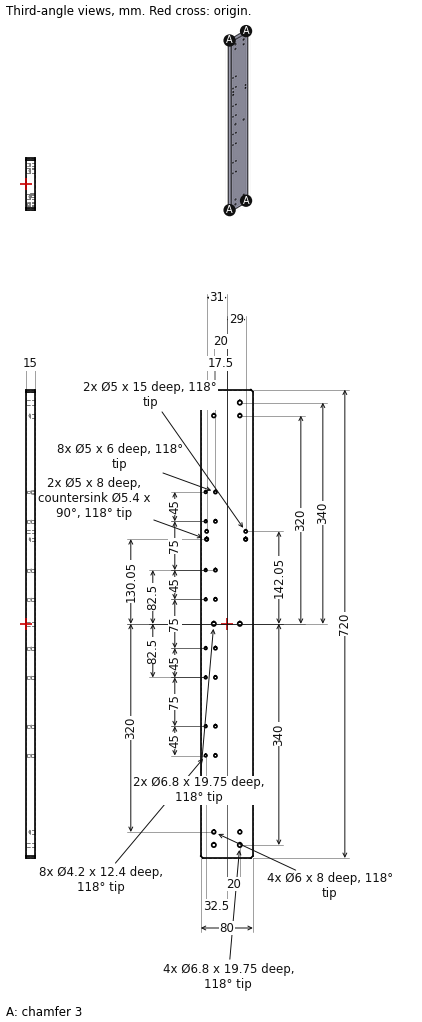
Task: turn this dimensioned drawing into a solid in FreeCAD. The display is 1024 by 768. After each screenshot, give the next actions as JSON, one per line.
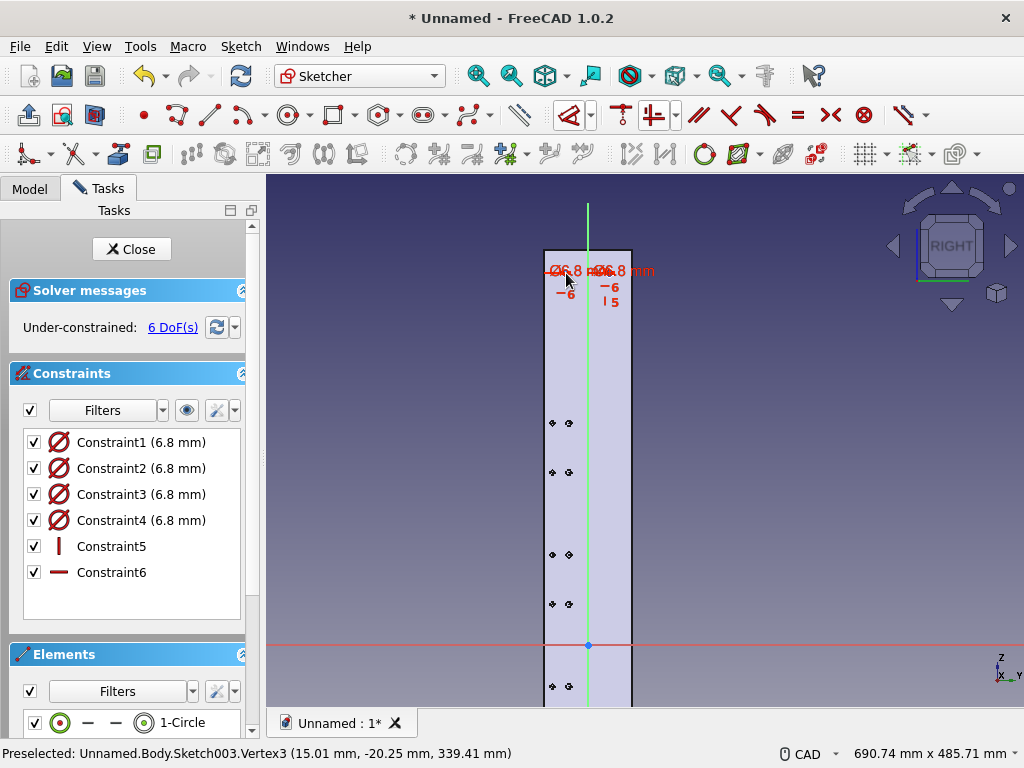
{"action": "left_click", "coordinate": [566, 273]}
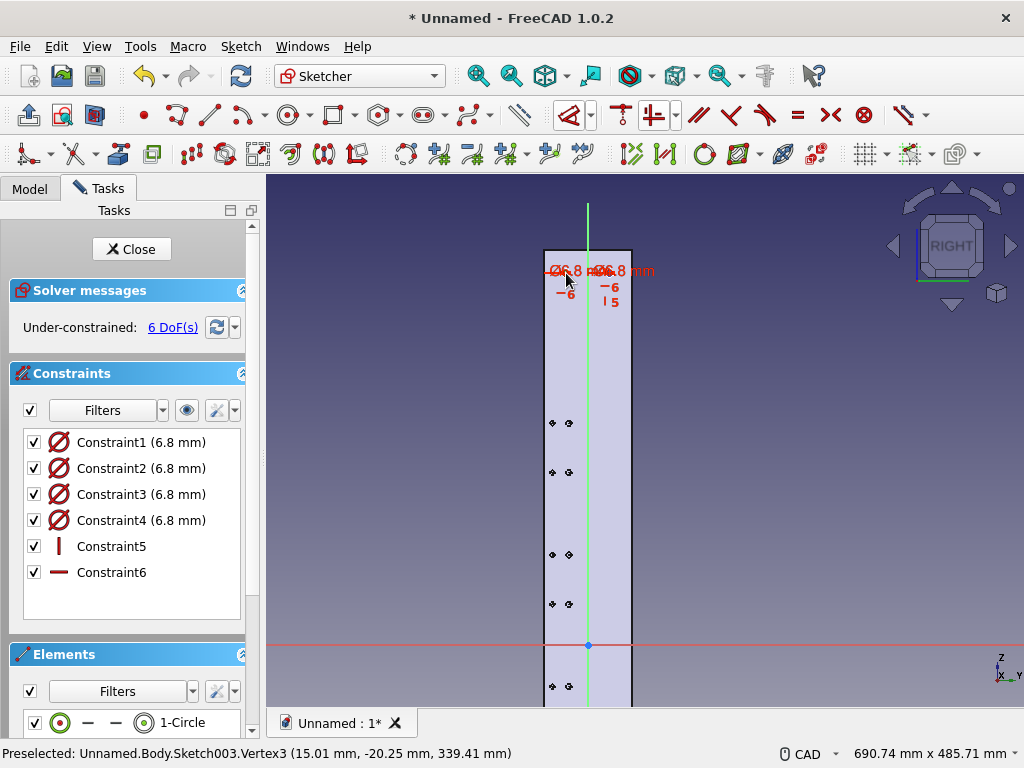
{"action": "scroll", "coordinate": [567, 273], "scroll_direction": "down", "scroll_amount": 4}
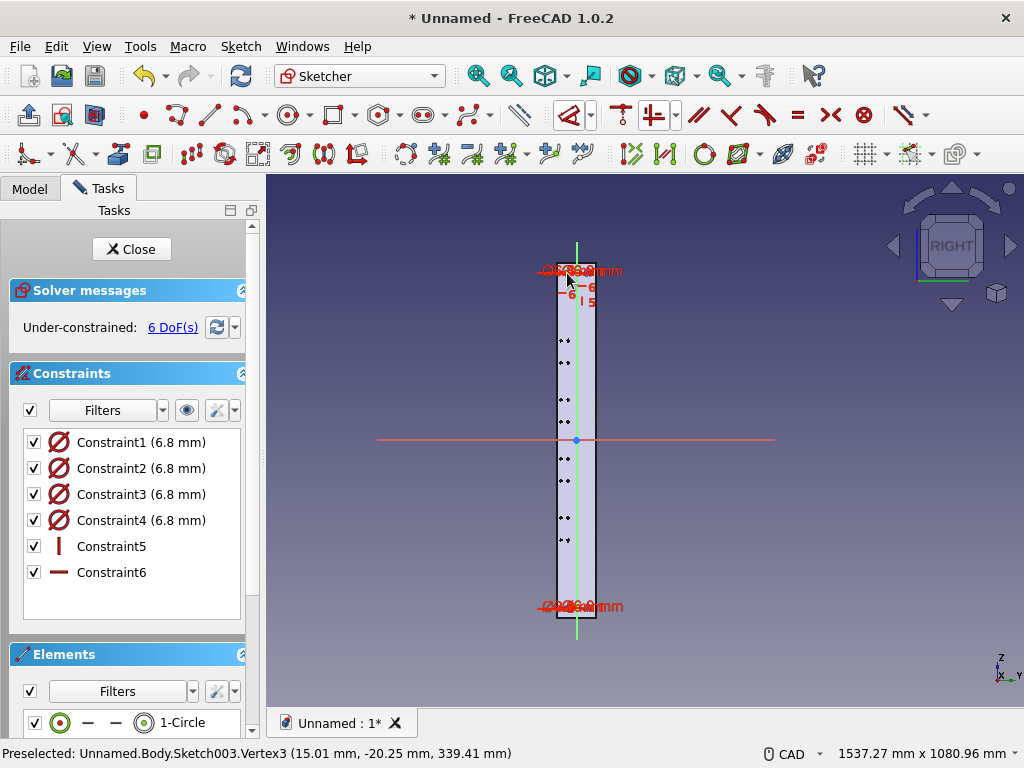
{"action": "left_click", "coordinate": [567, 609]}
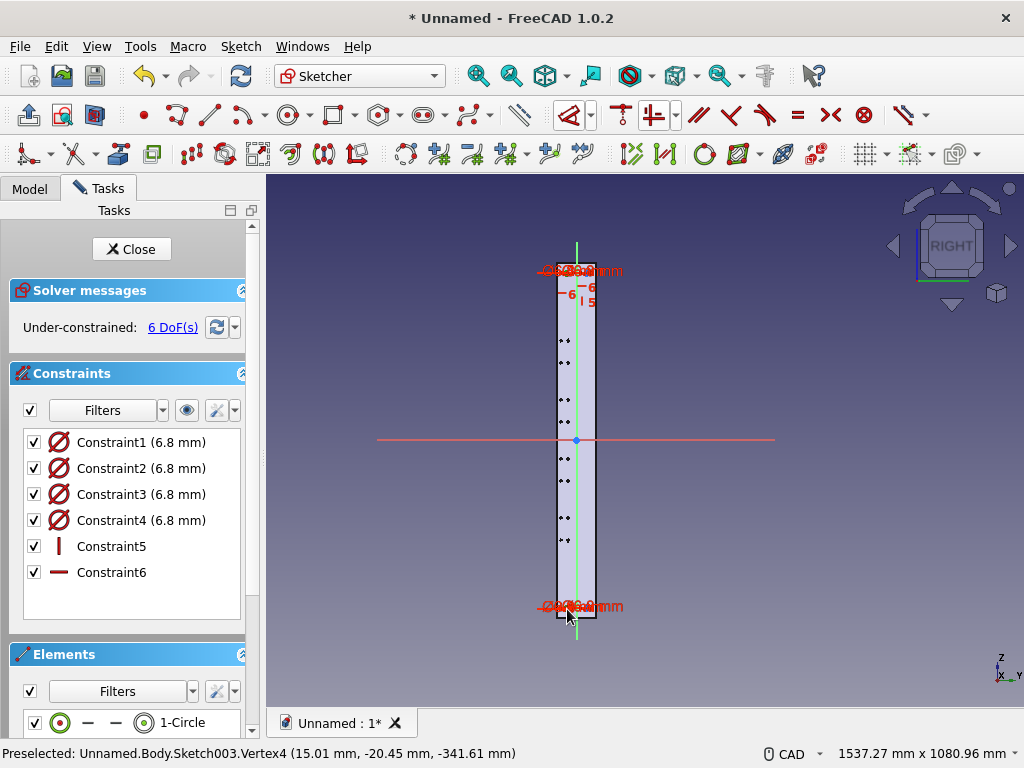
{"action": "left_click", "coordinate": [676, 116]}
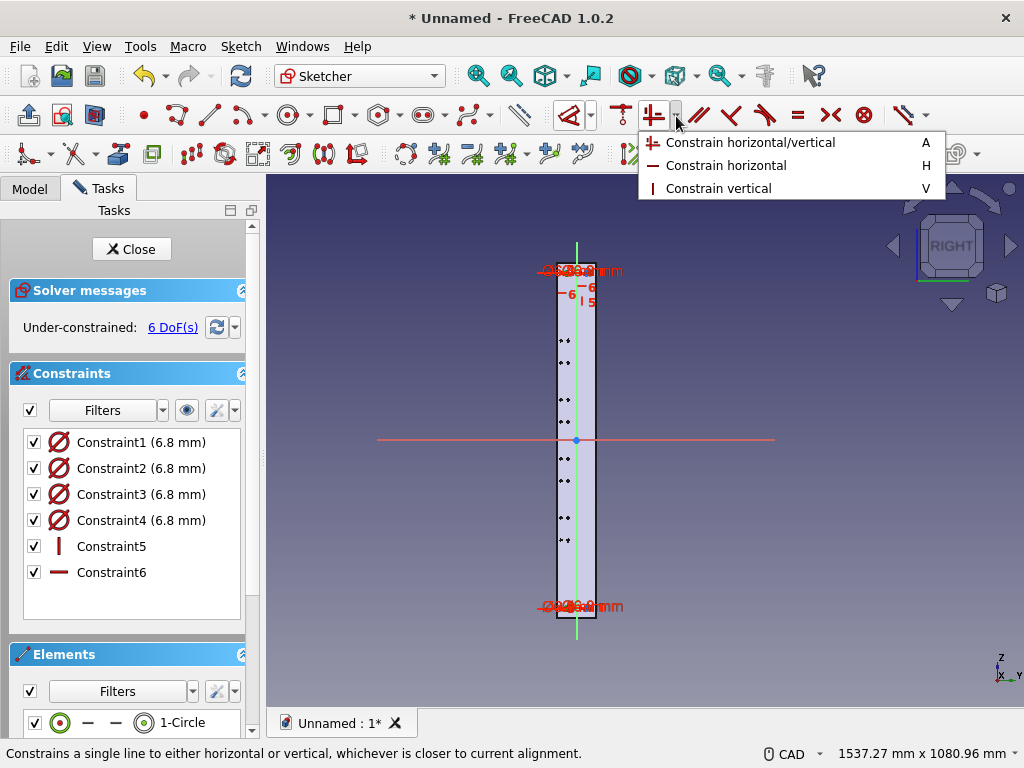
{"action": "left_click", "coordinate": [792, 188]}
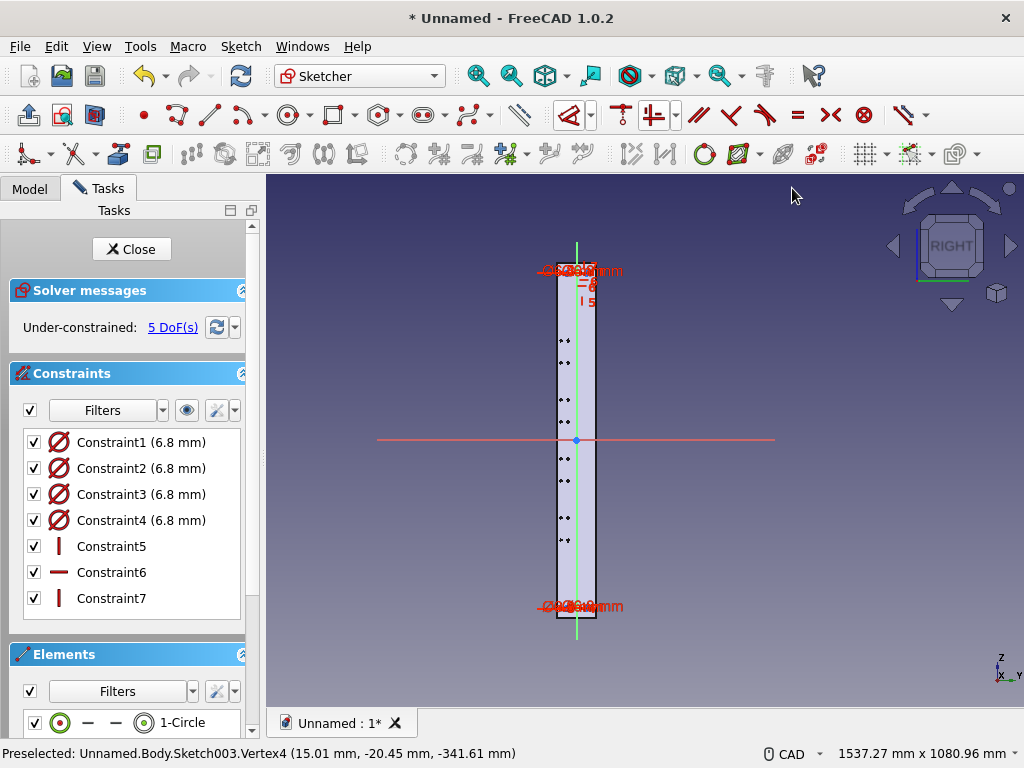
{"action": "scroll", "coordinate": [586, 608], "scroll_direction": "up", "scroll_amount": 4}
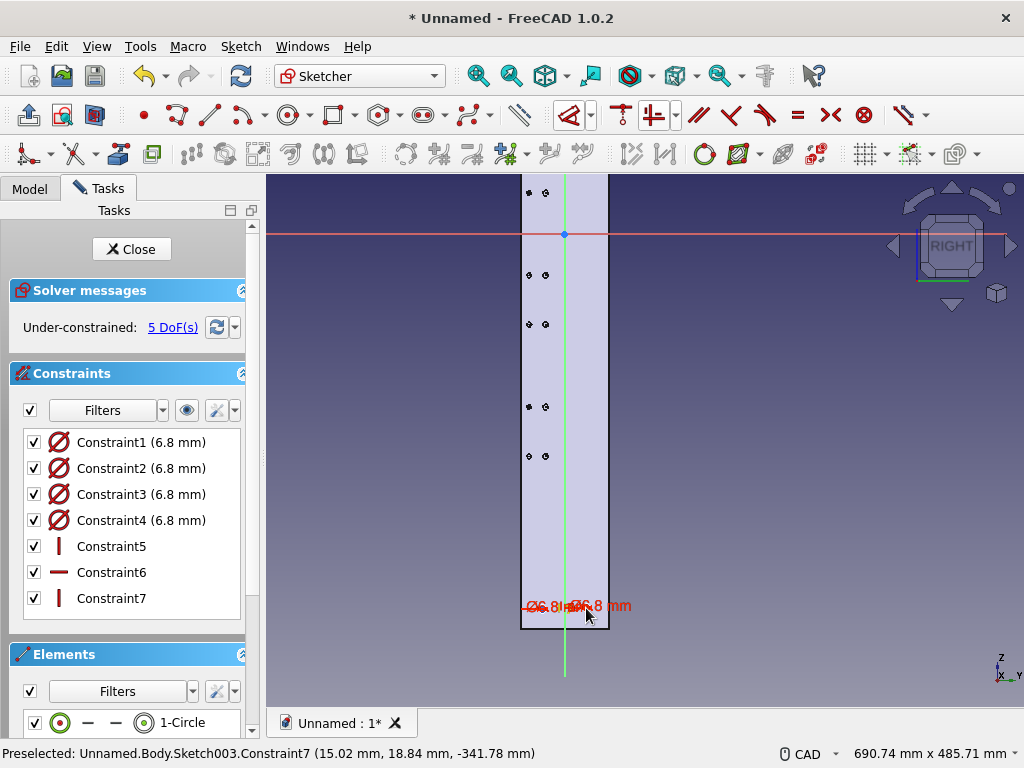
{"action": "left_click", "coordinate": [586, 608]}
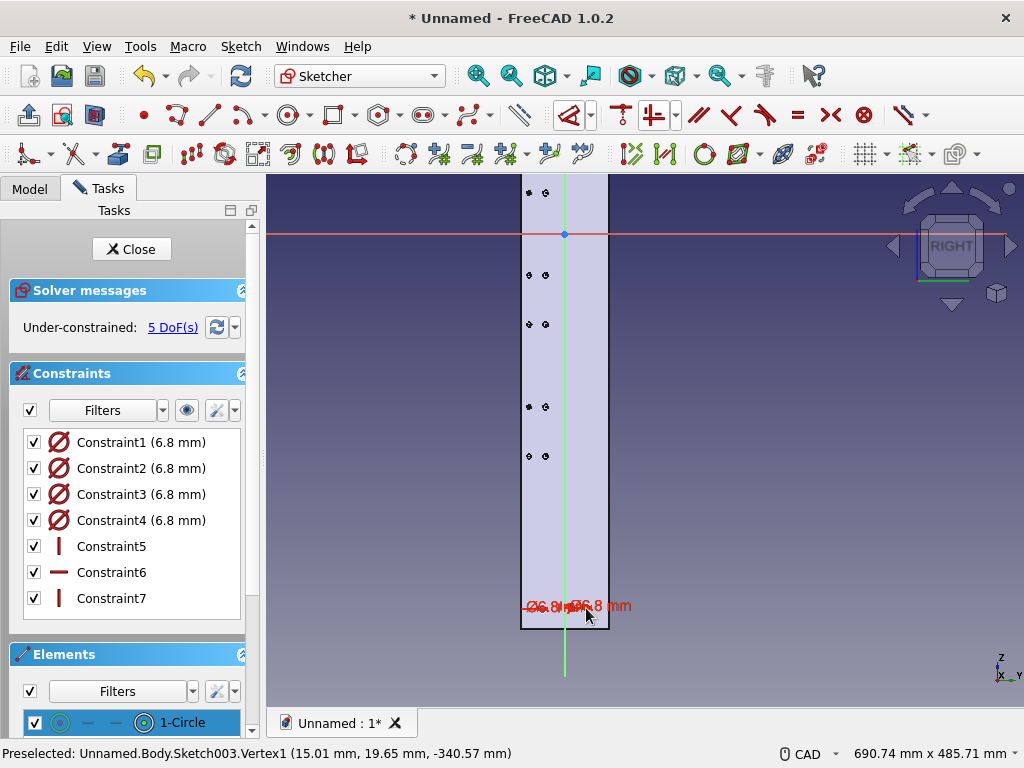
{"action": "left_click", "coordinate": [543, 609]}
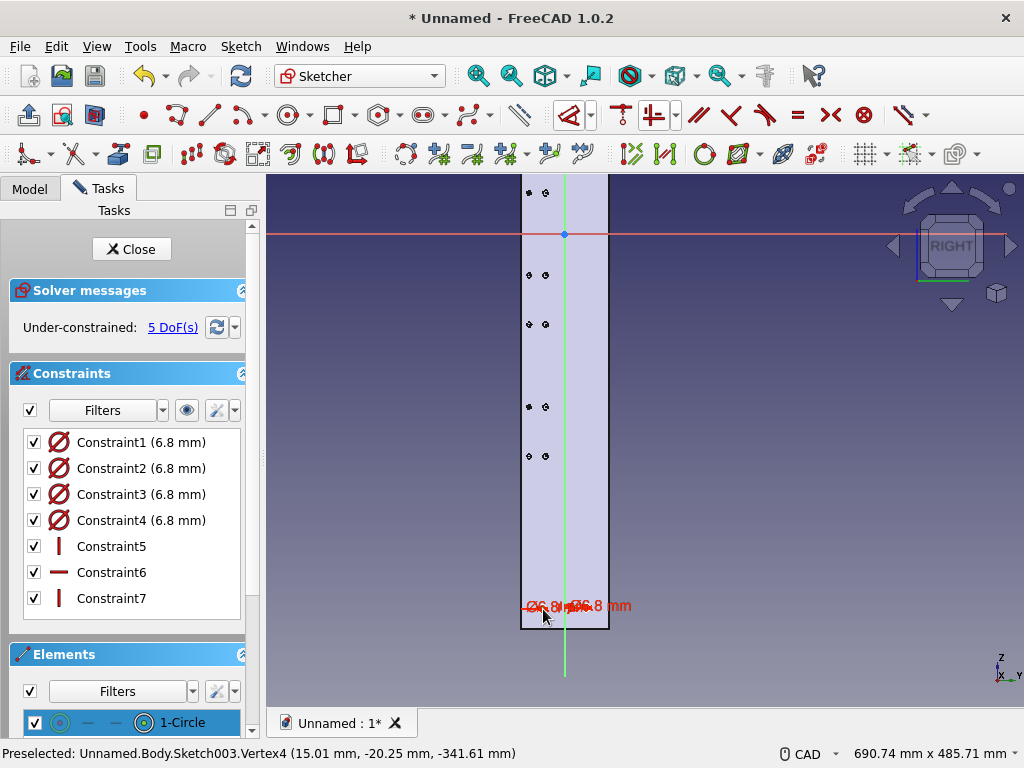
{"action": "left_click", "coordinate": [676, 116]}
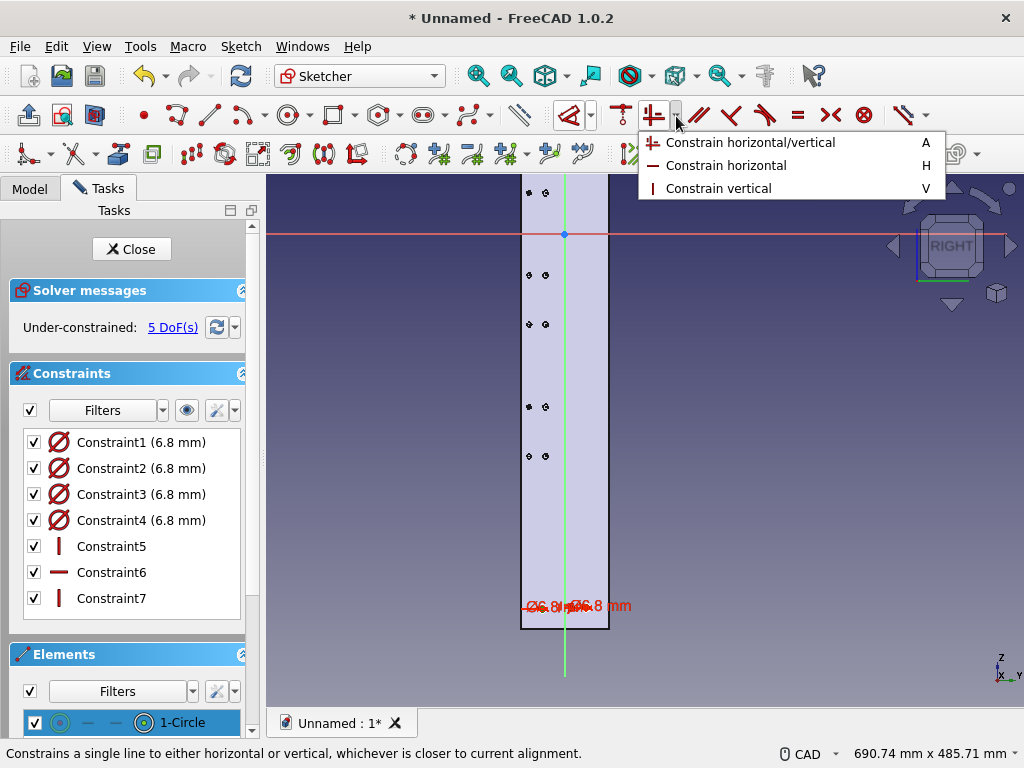
{"action": "left_click", "coordinate": [792, 166]}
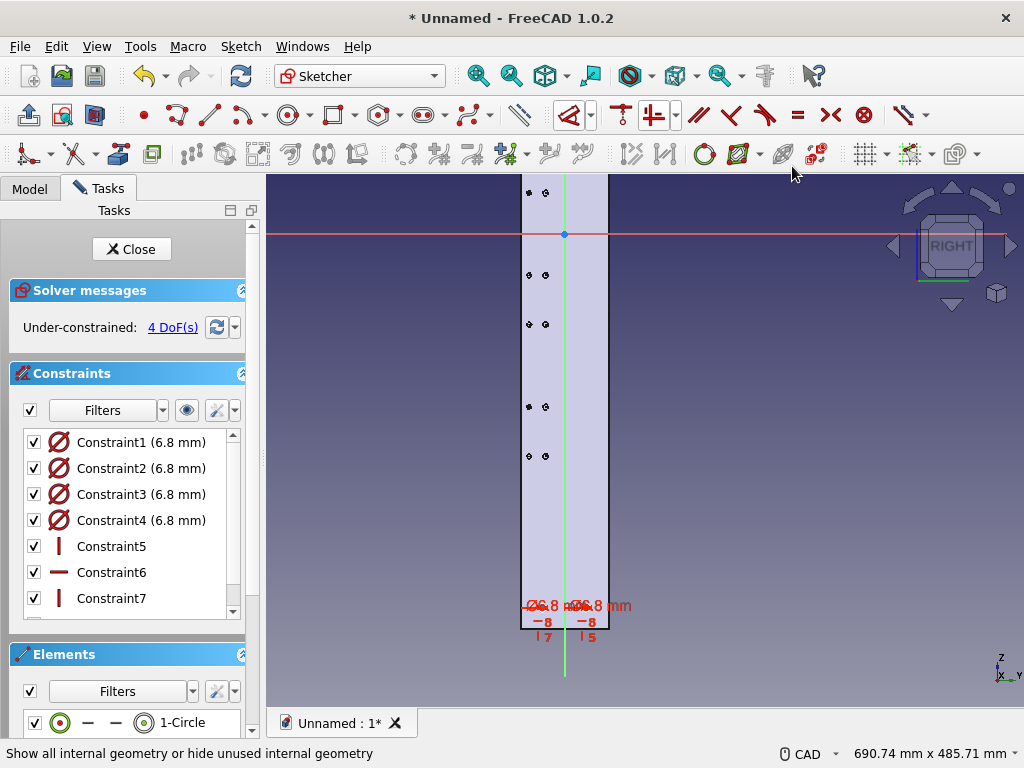
{"action": "scroll", "coordinate": [586, 608], "scroll_direction": "up", "scroll_amount": 3}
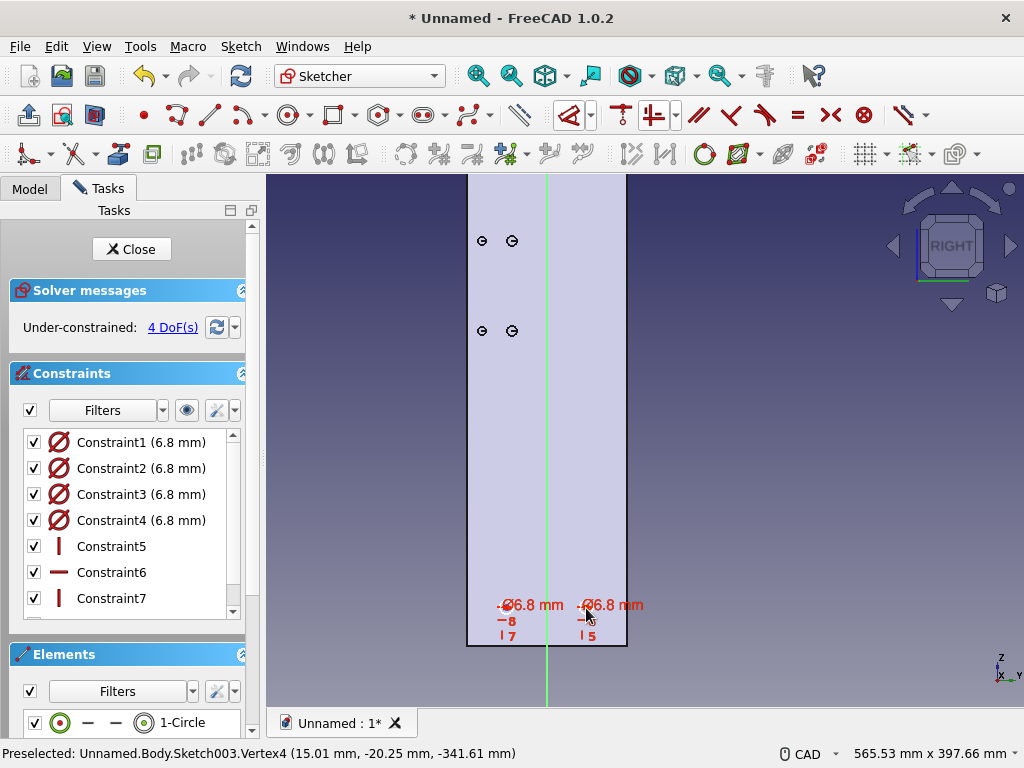
{"action": "left_click", "coordinate": [586, 607]}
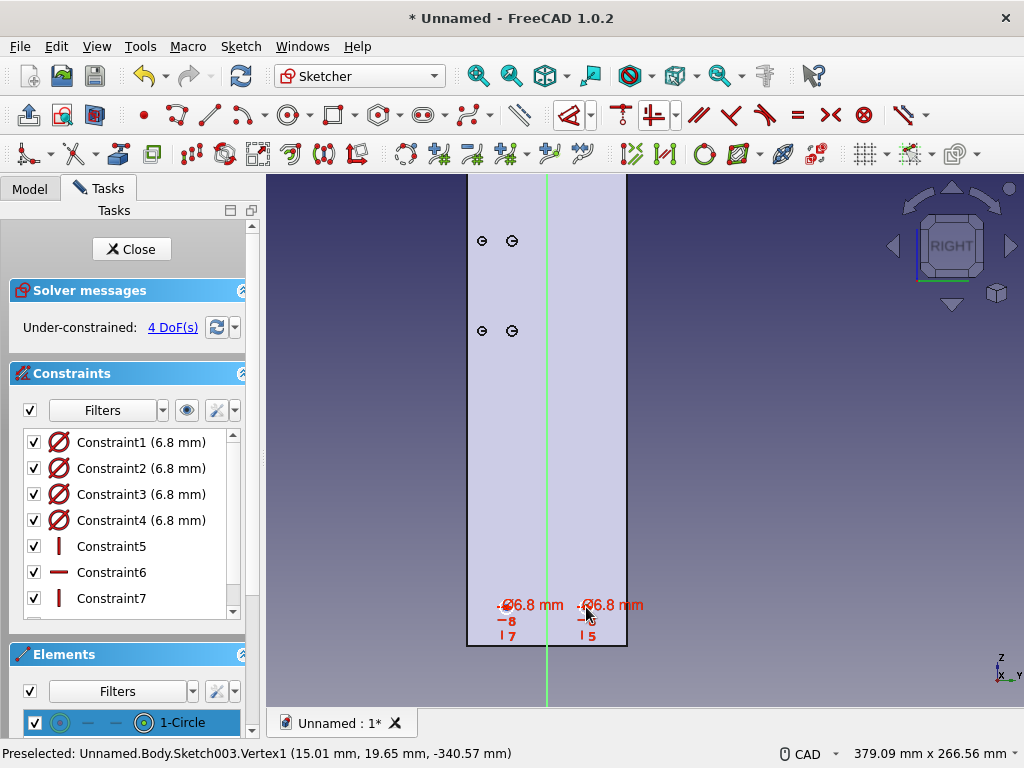
{"action": "key", "text": "l"}